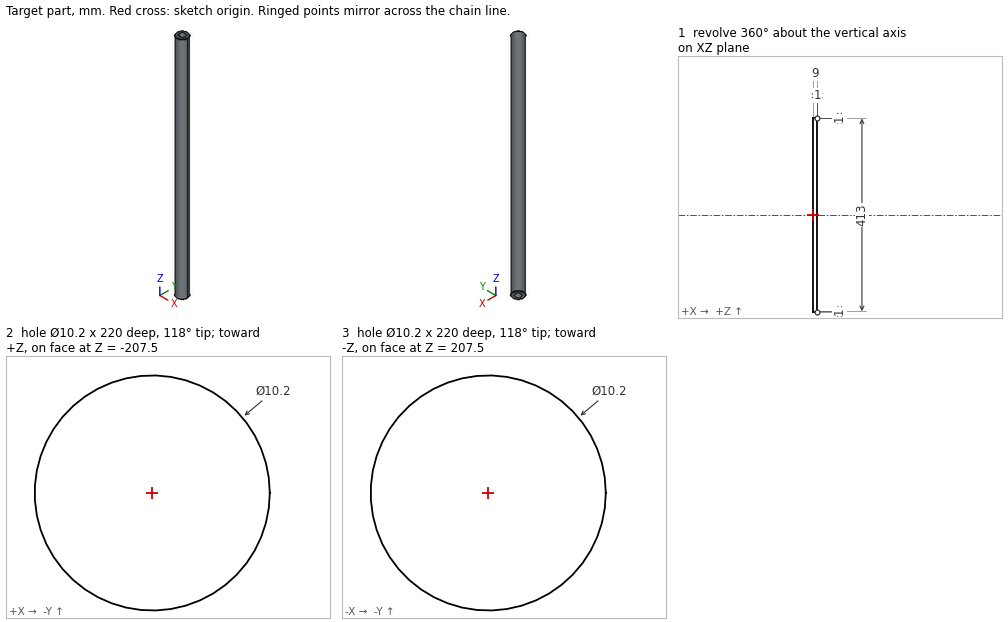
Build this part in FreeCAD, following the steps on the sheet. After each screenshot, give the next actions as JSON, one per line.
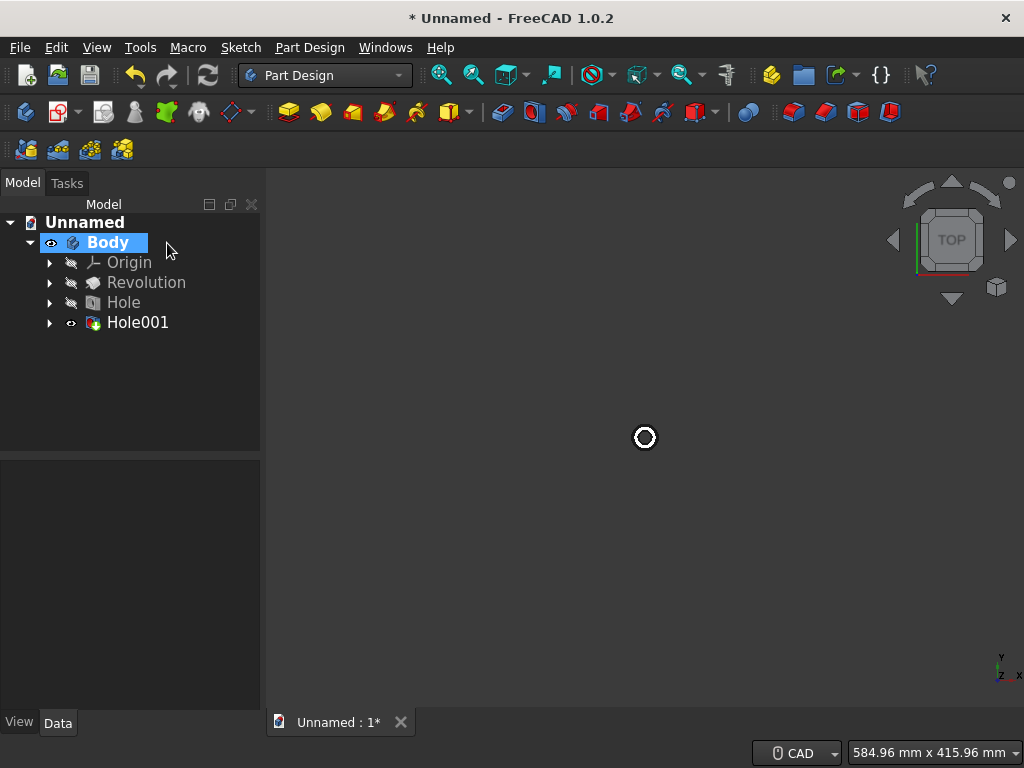
{"action": "key", "text": "0"}